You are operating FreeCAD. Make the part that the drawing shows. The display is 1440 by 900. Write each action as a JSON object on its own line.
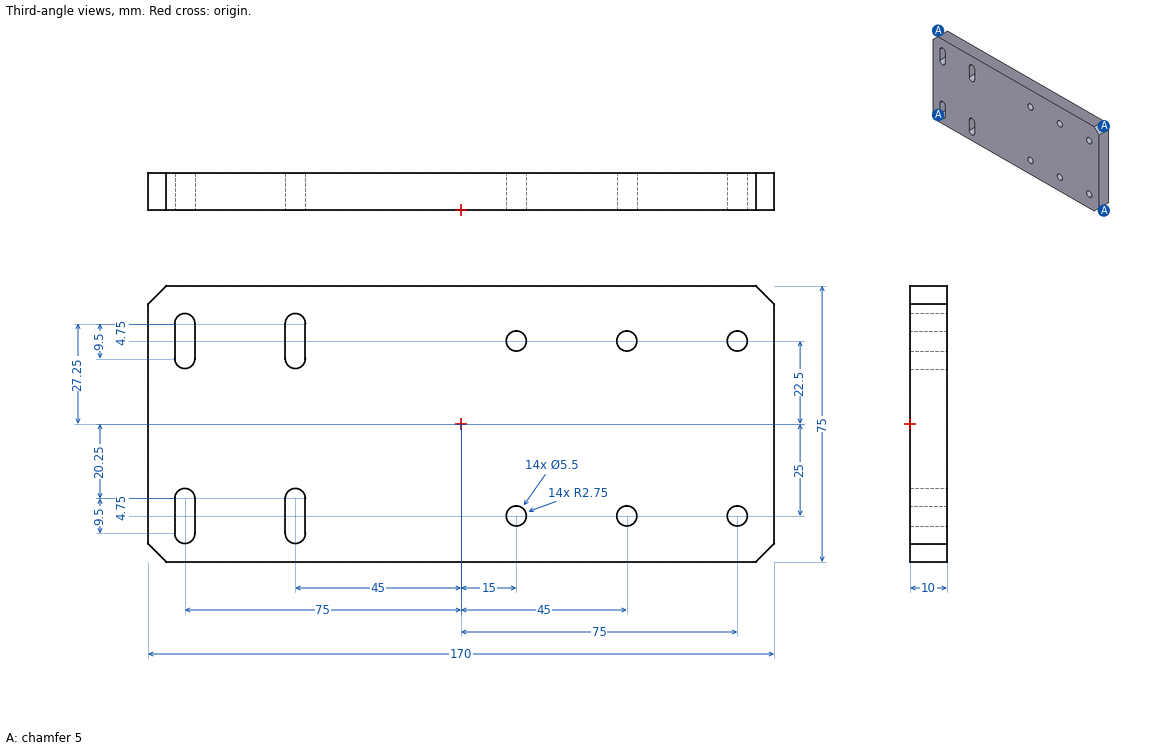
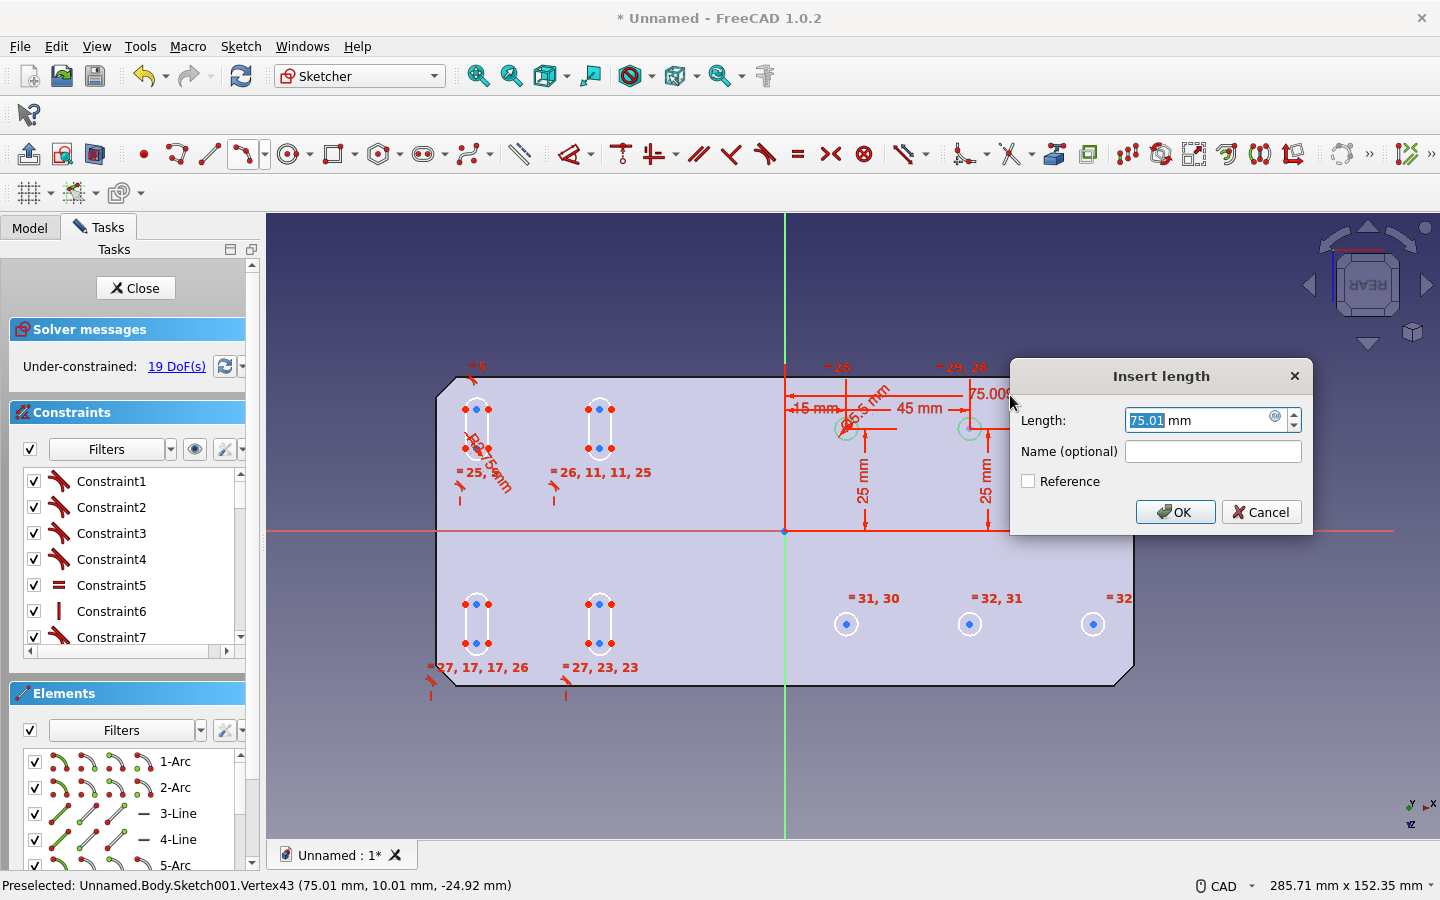
{"action": "type", "text": "75"}
{"action": "key", "text": "Return"}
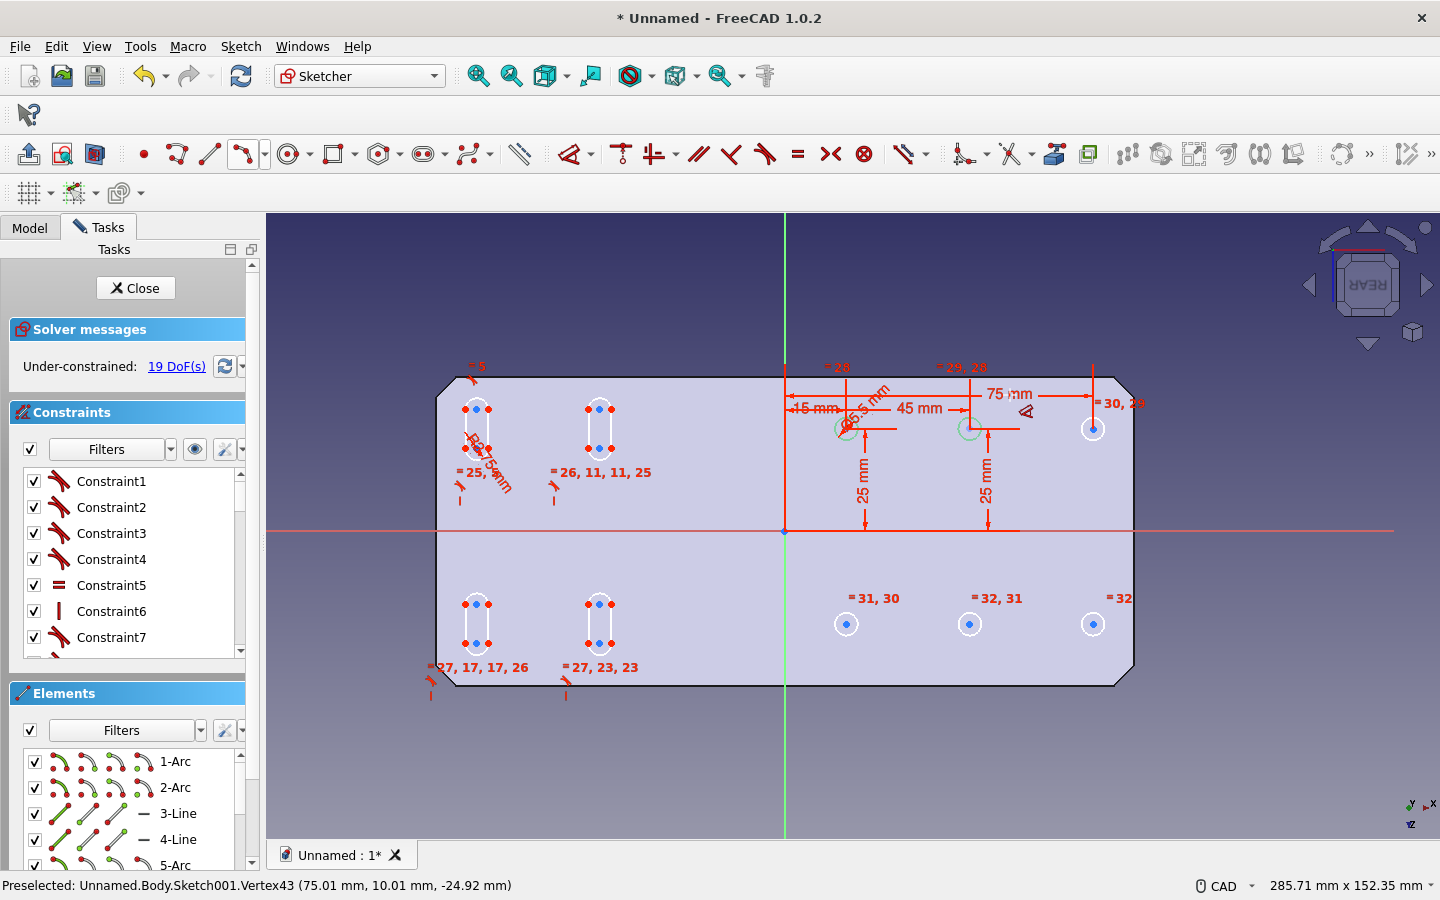
{"action": "left_click", "coordinate": [1093, 429]}
{"action": "left_click", "coordinate": [1127, 480]}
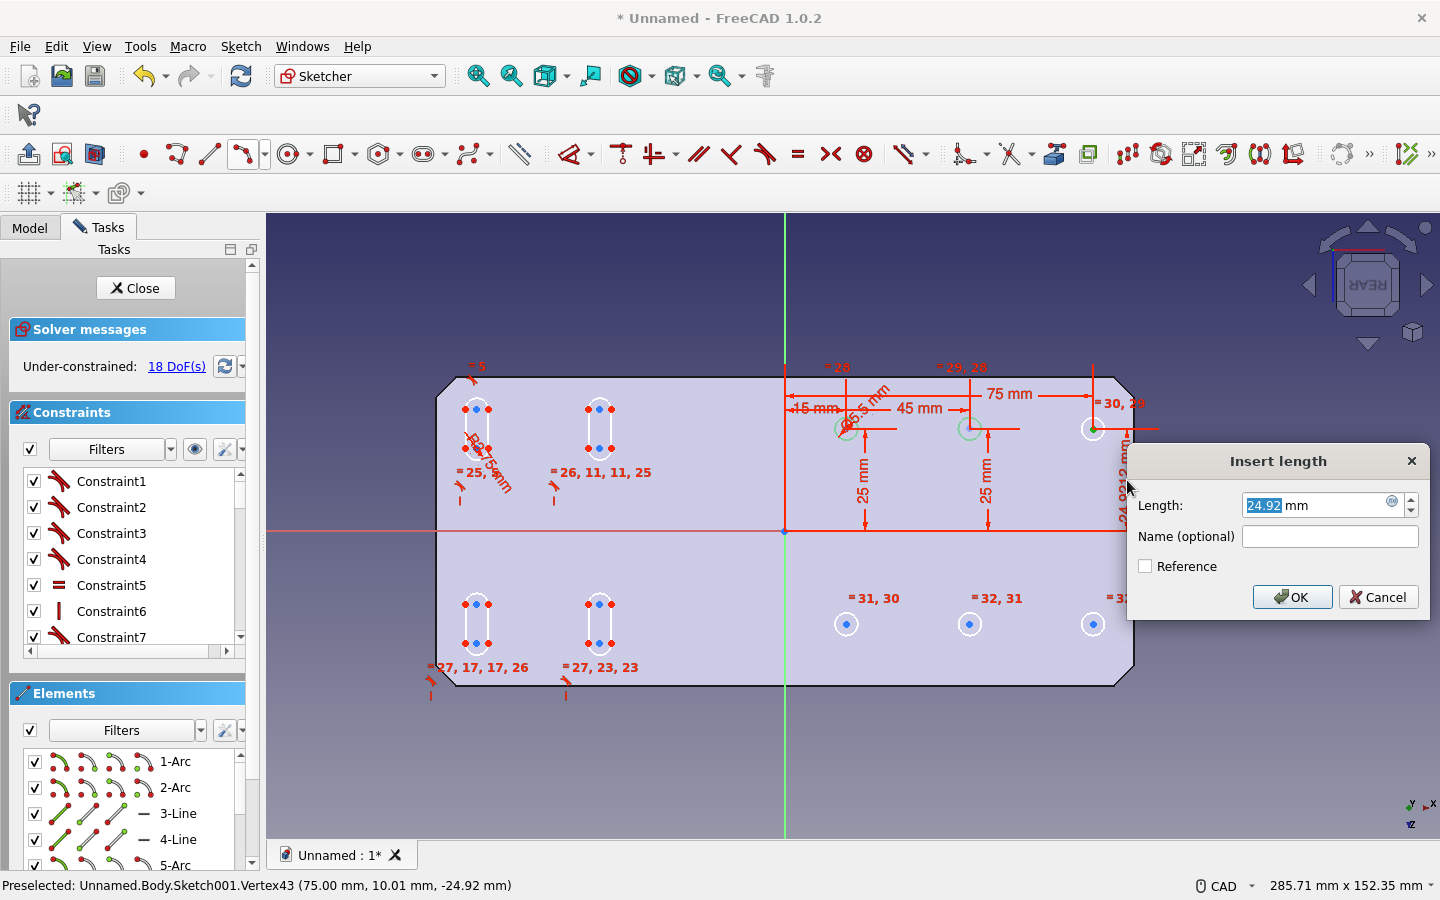
{"action": "type", "text": "25"}
{"action": "key", "text": "Return"}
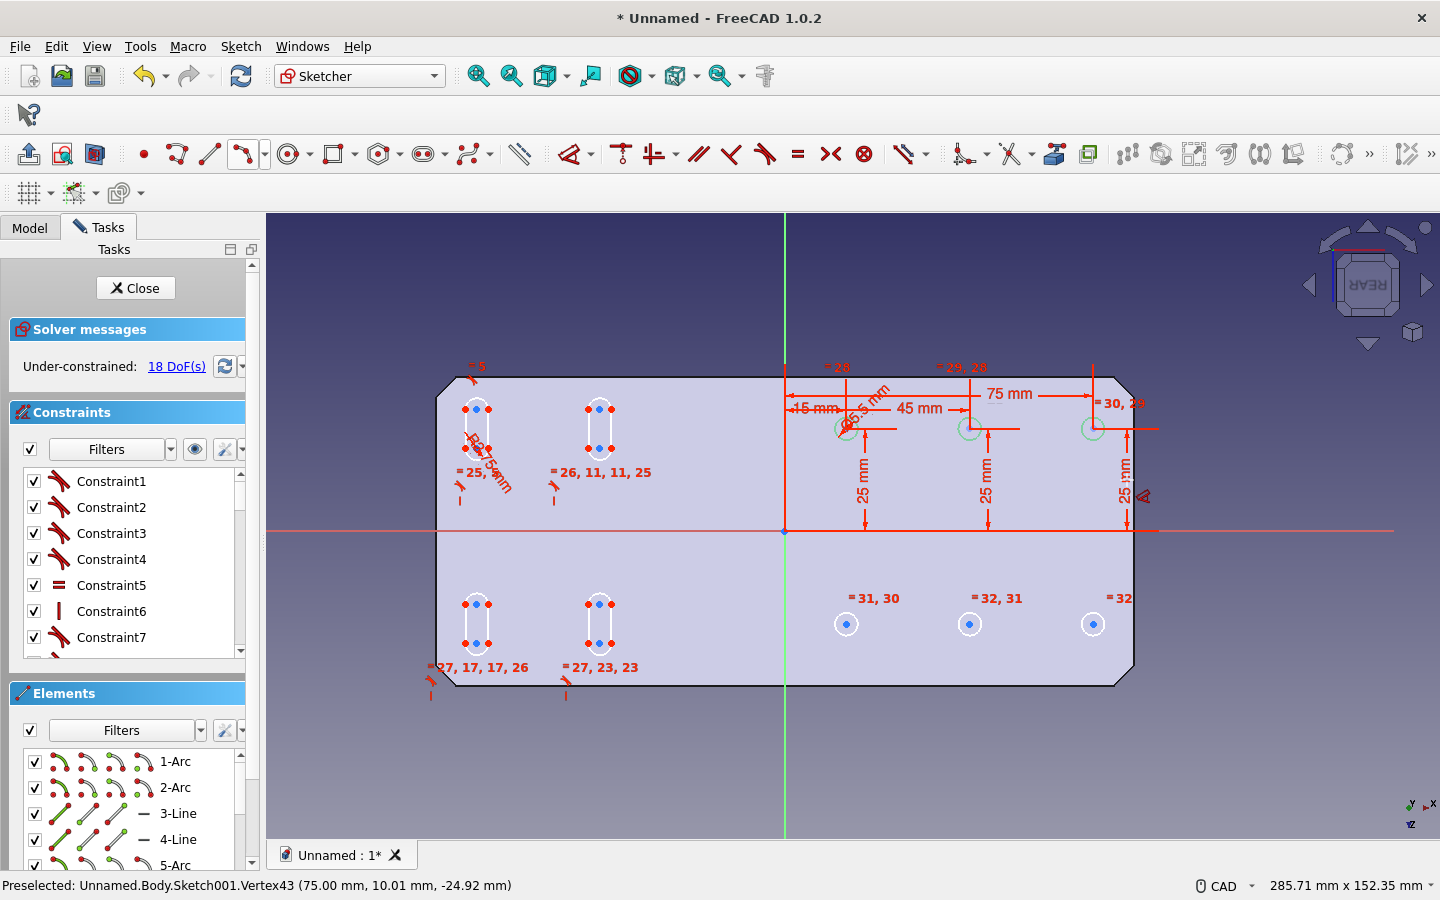
{"action": "left_click", "coordinate": [846, 624]}
{"action": "left_click", "coordinate": [816, 658]}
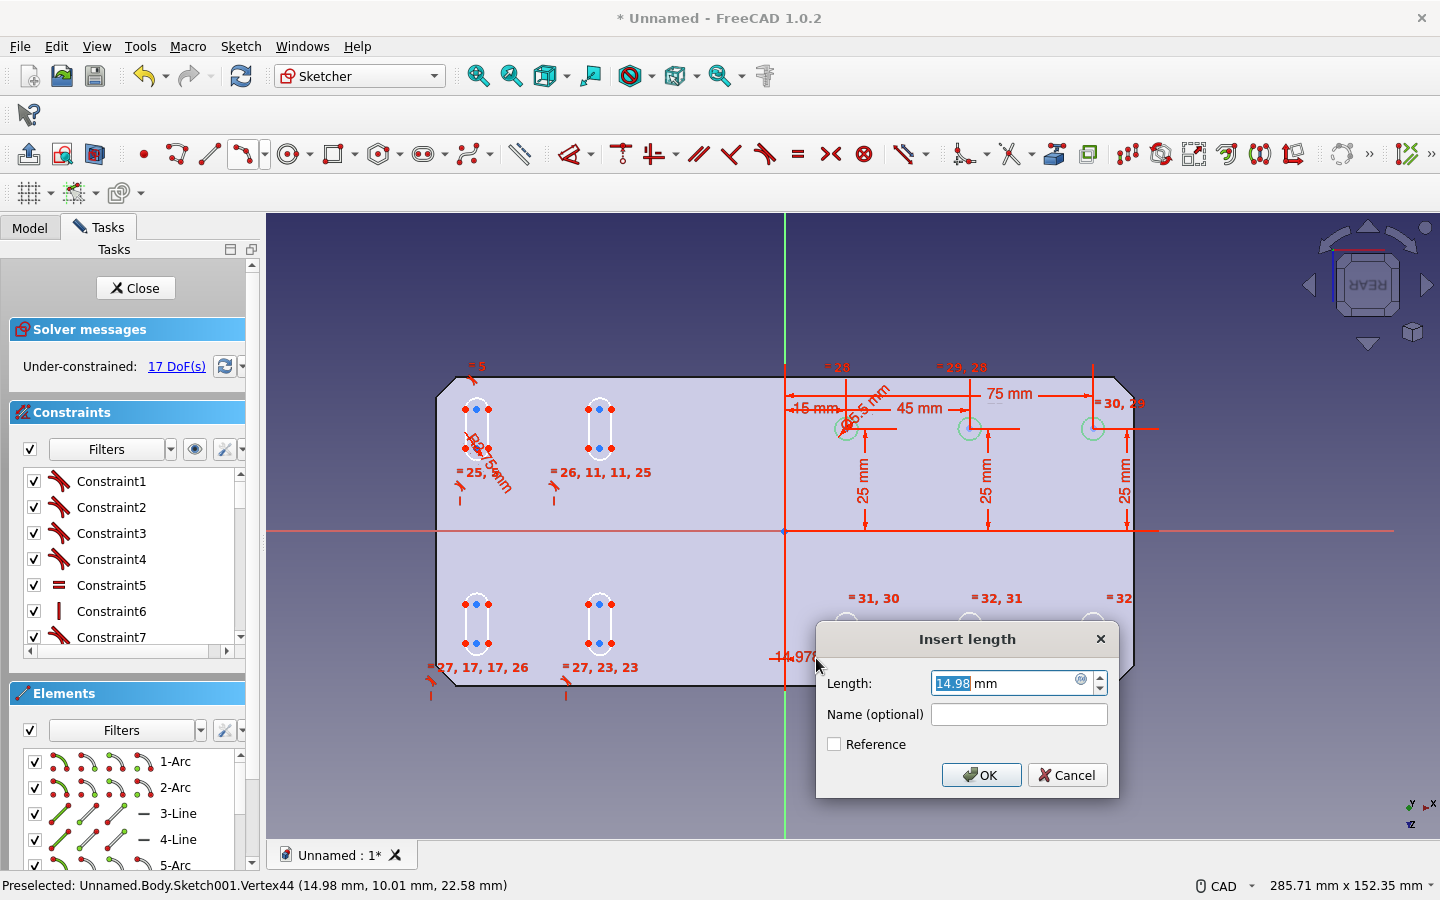
{"action": "type", "text": "15"}
{"action": "key", "text": "Return"}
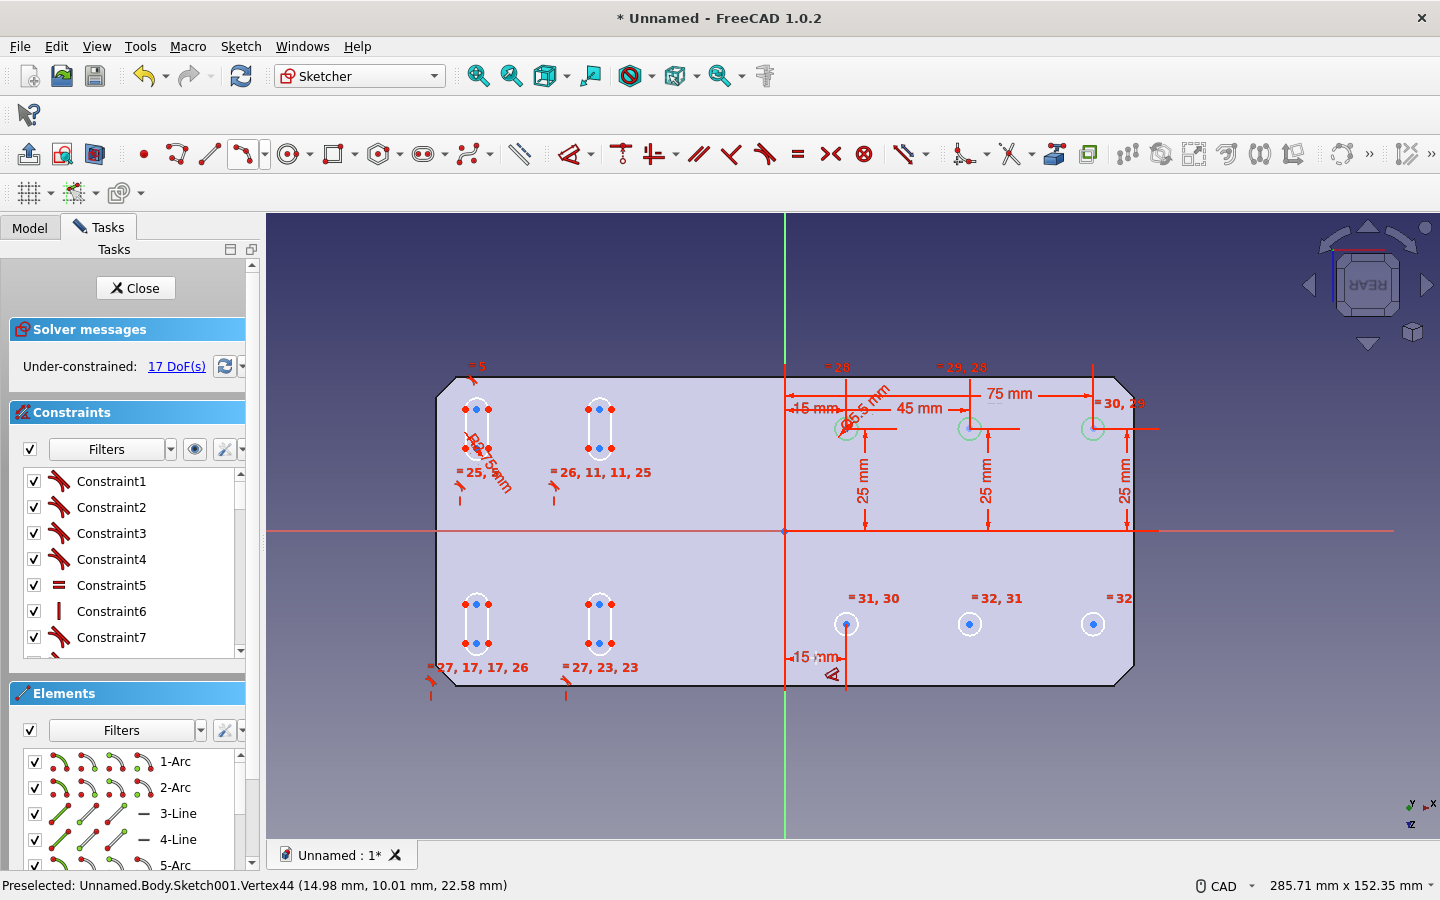
{"action": "left_click", "coordinate": [970, 624]}
{"action": "left_click", "coordinate": [920, 658]}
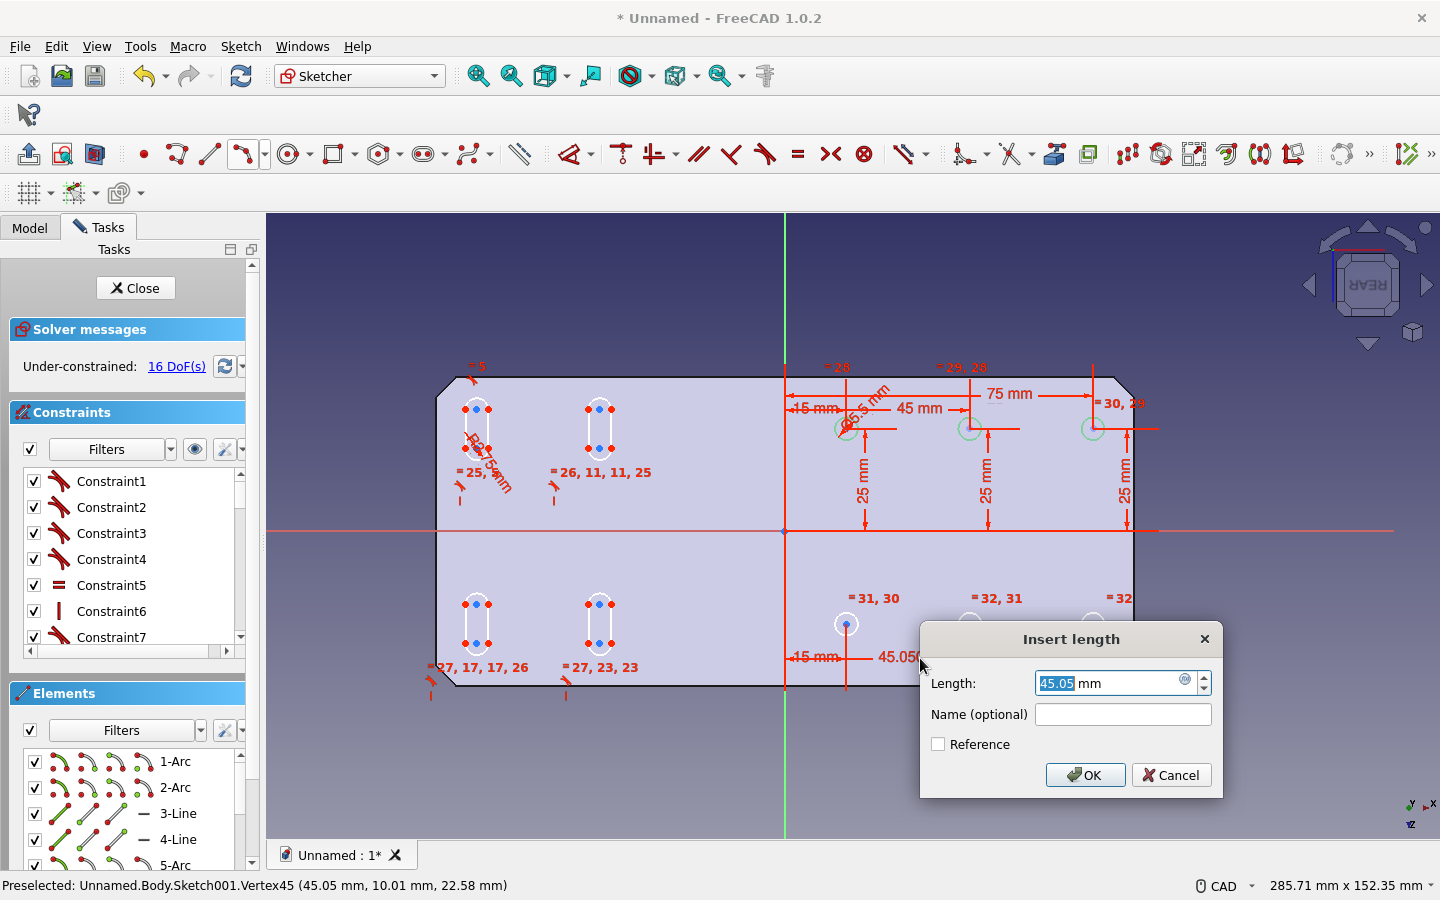
{"action": "type", "text": "45"}
{"action": "key", "text": "Return"}